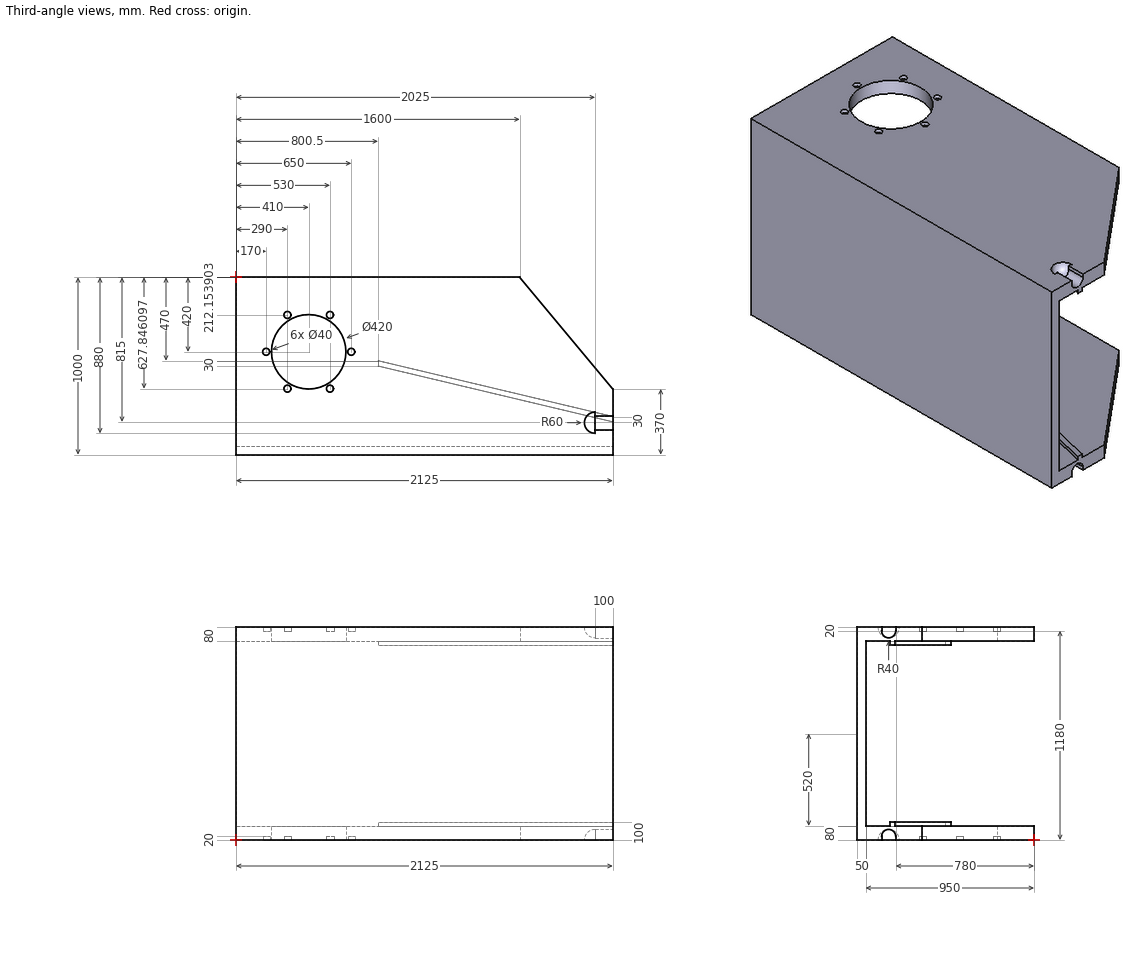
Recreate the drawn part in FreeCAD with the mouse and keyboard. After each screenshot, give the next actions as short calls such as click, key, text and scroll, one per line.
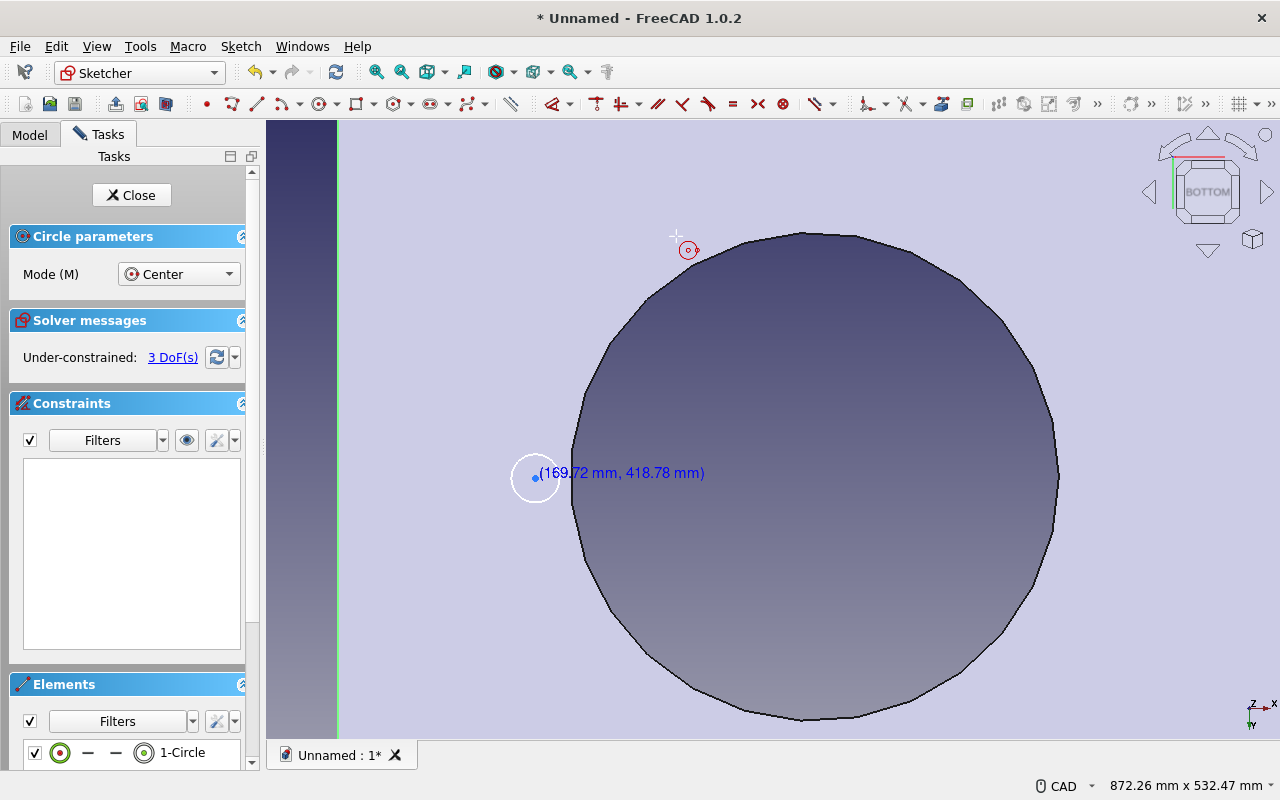
click(675, 235)
click(692, 219)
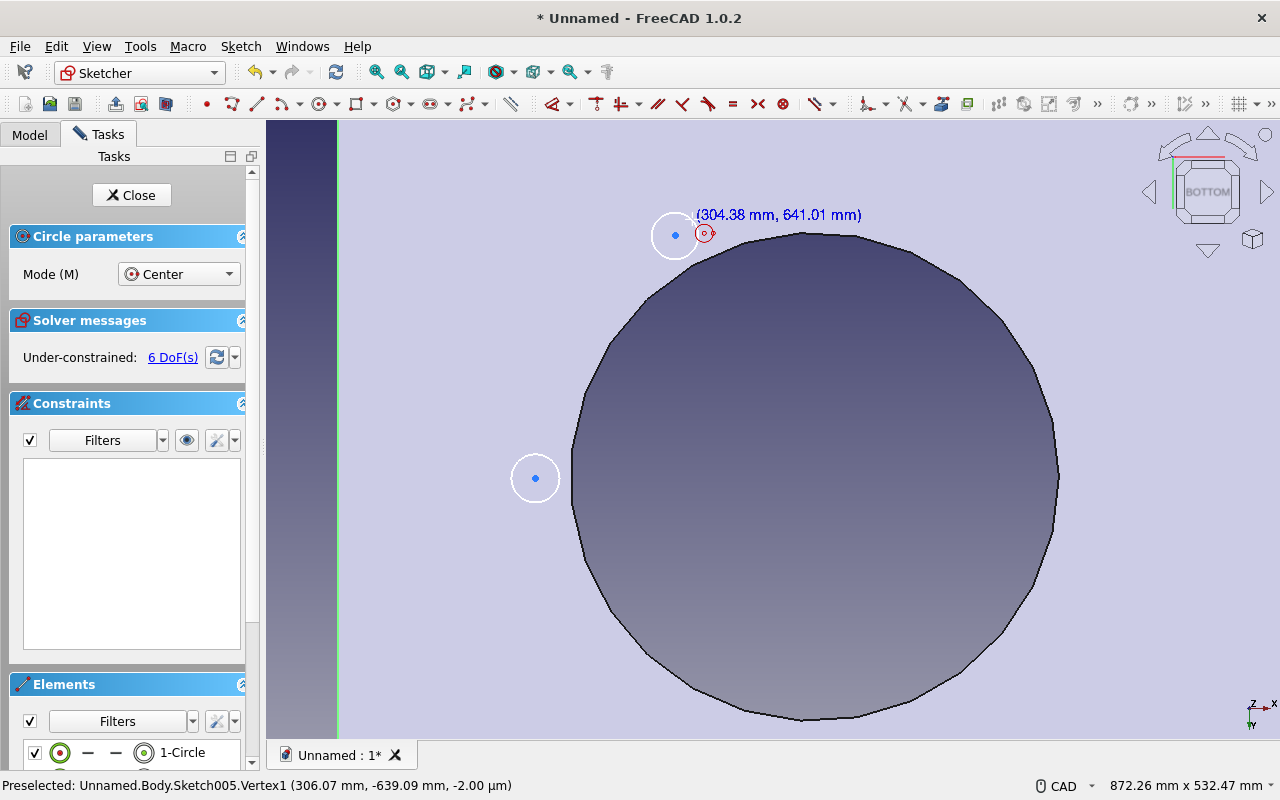
click(954, 235)
click(971, 219)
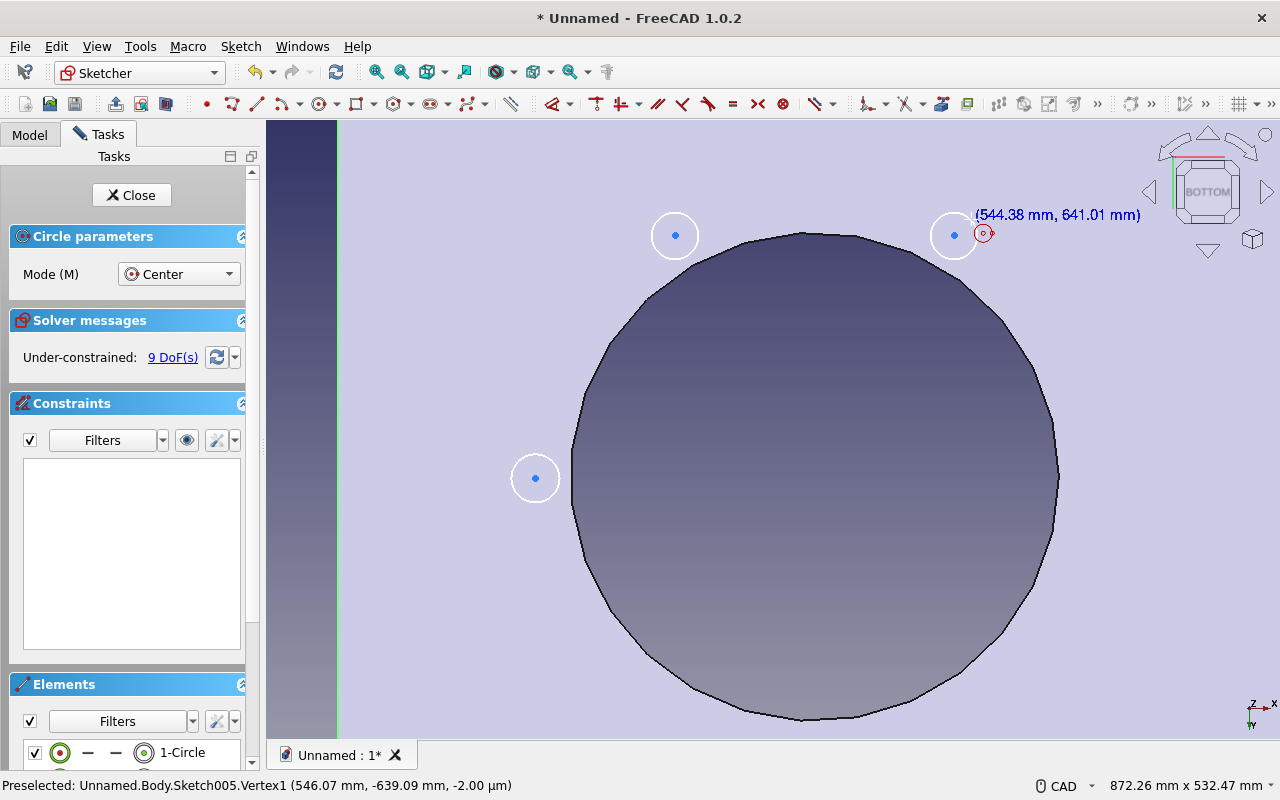
click(1094, 477)
click(1110, 460)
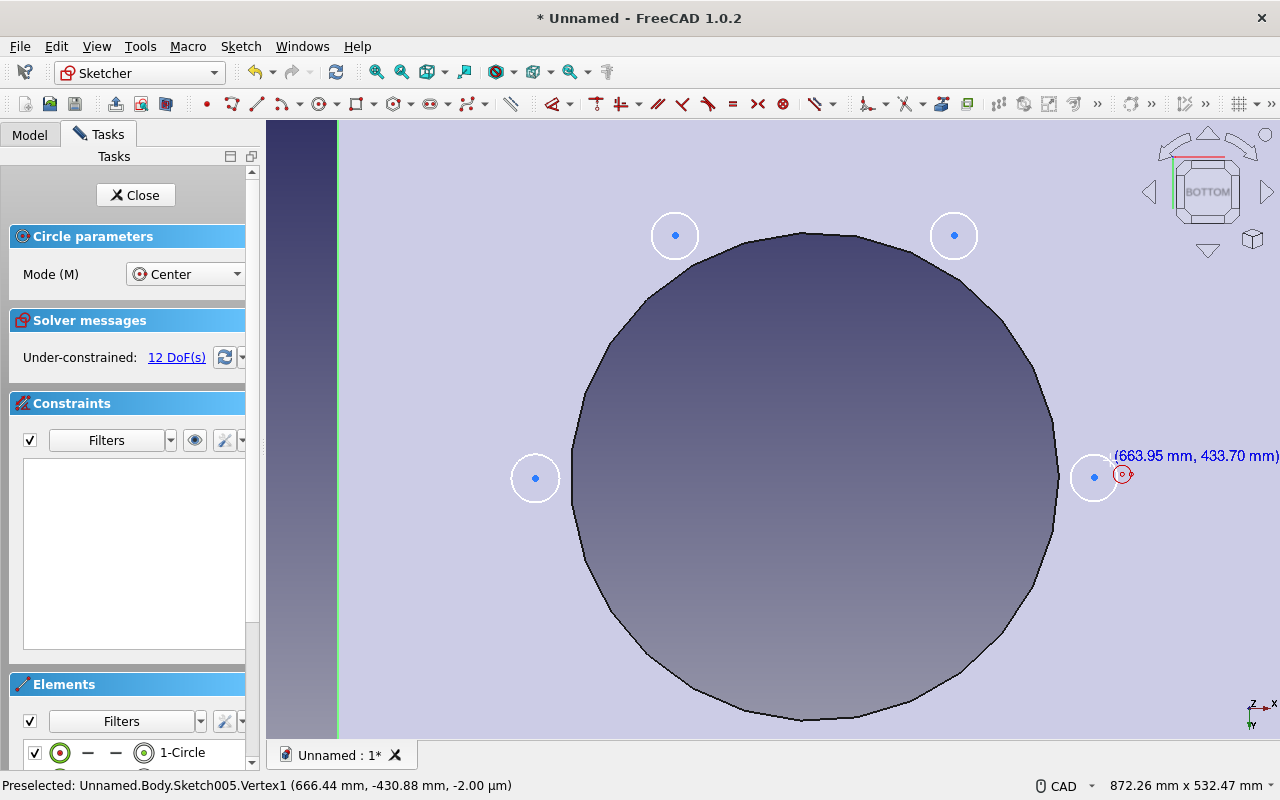
scroll(676, 236, down, 3)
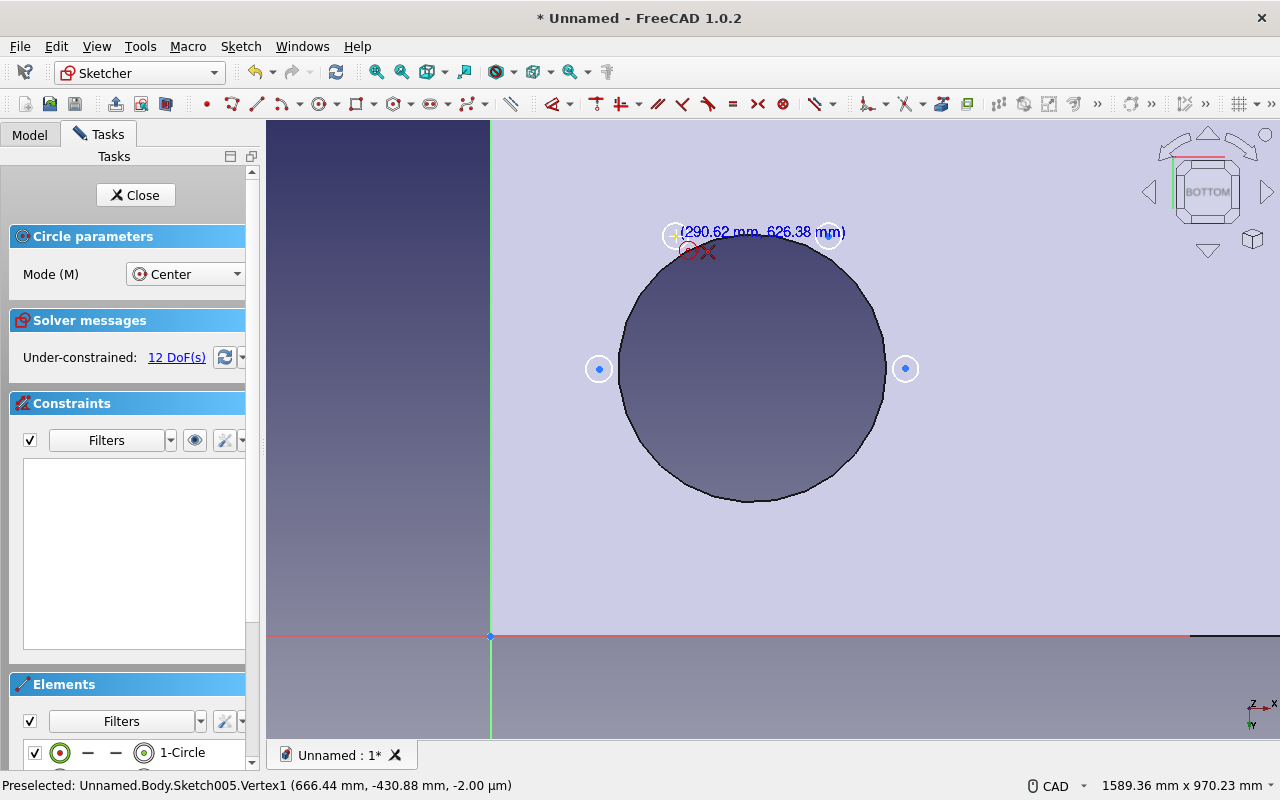
scroll(676, 501, up, 3)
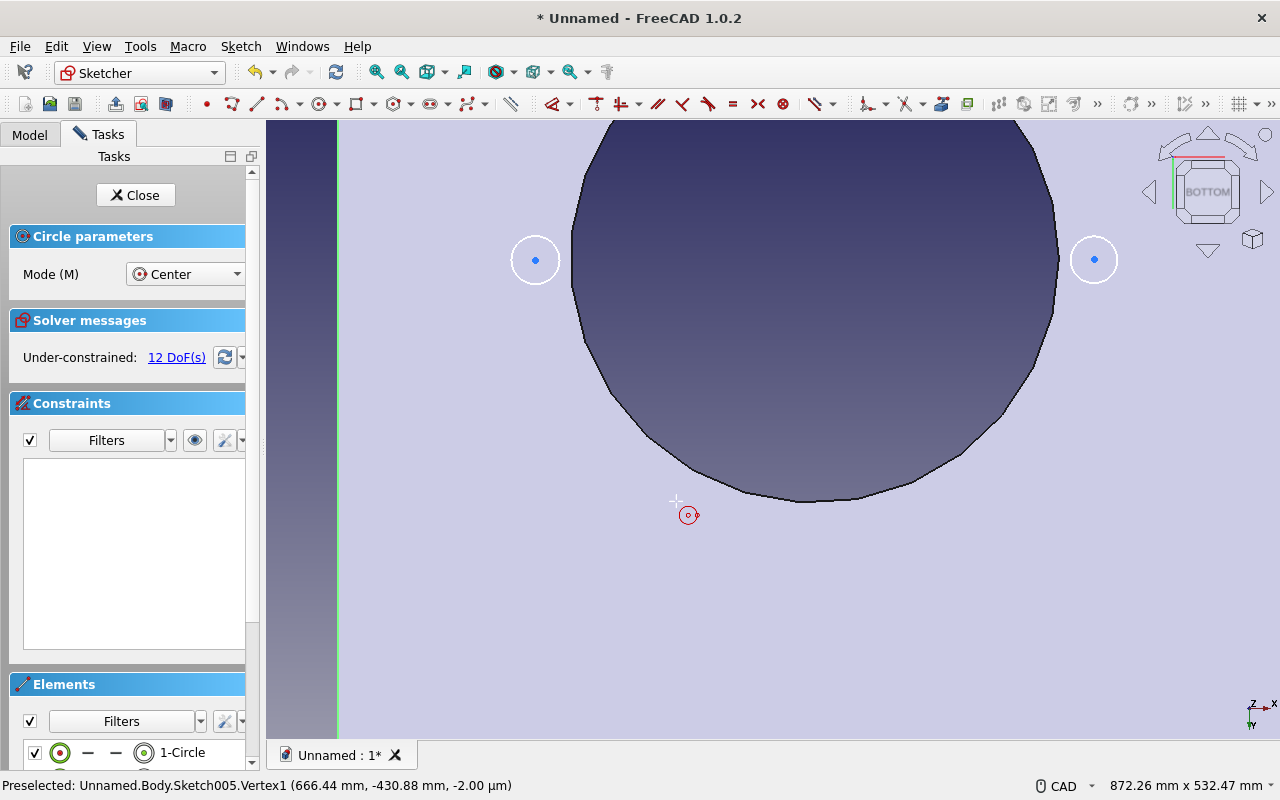
click(675, 500)
click(692, 484)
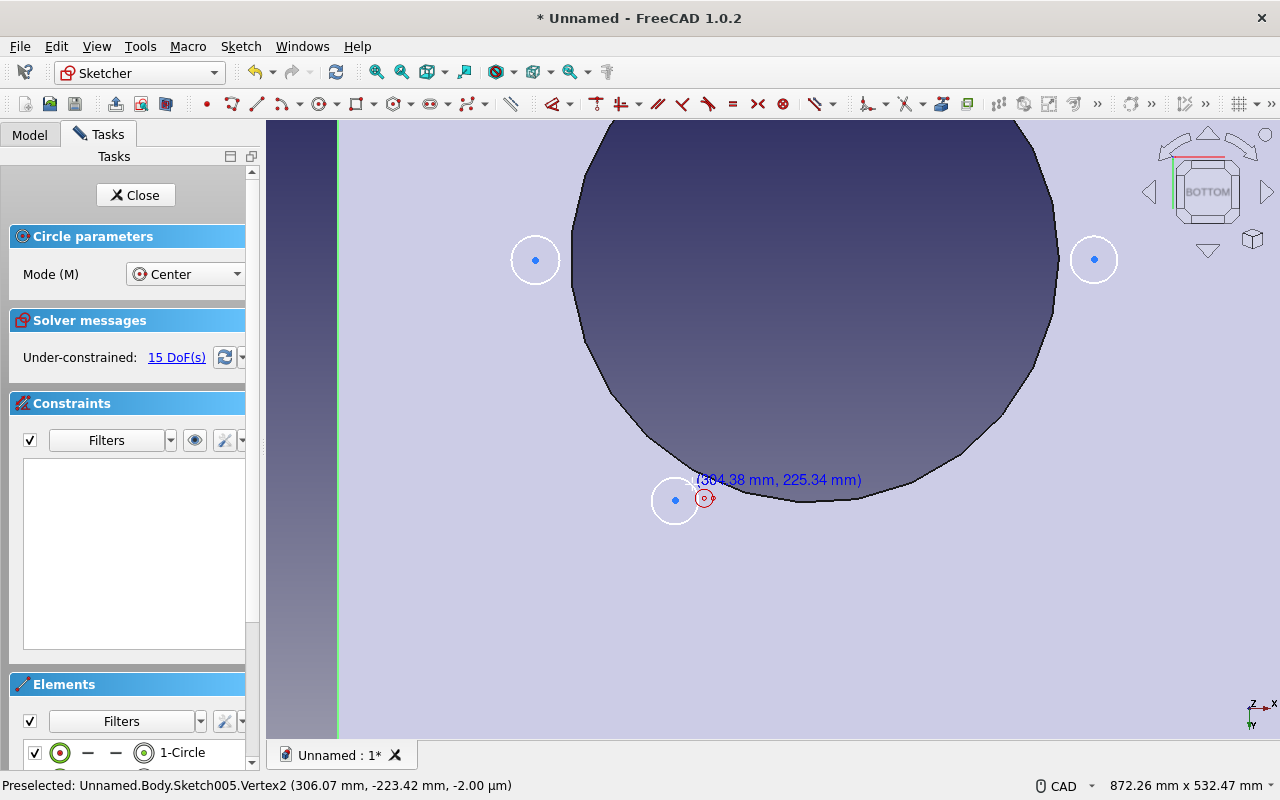
click(954, 500)
click(971, 484)
key(Escape)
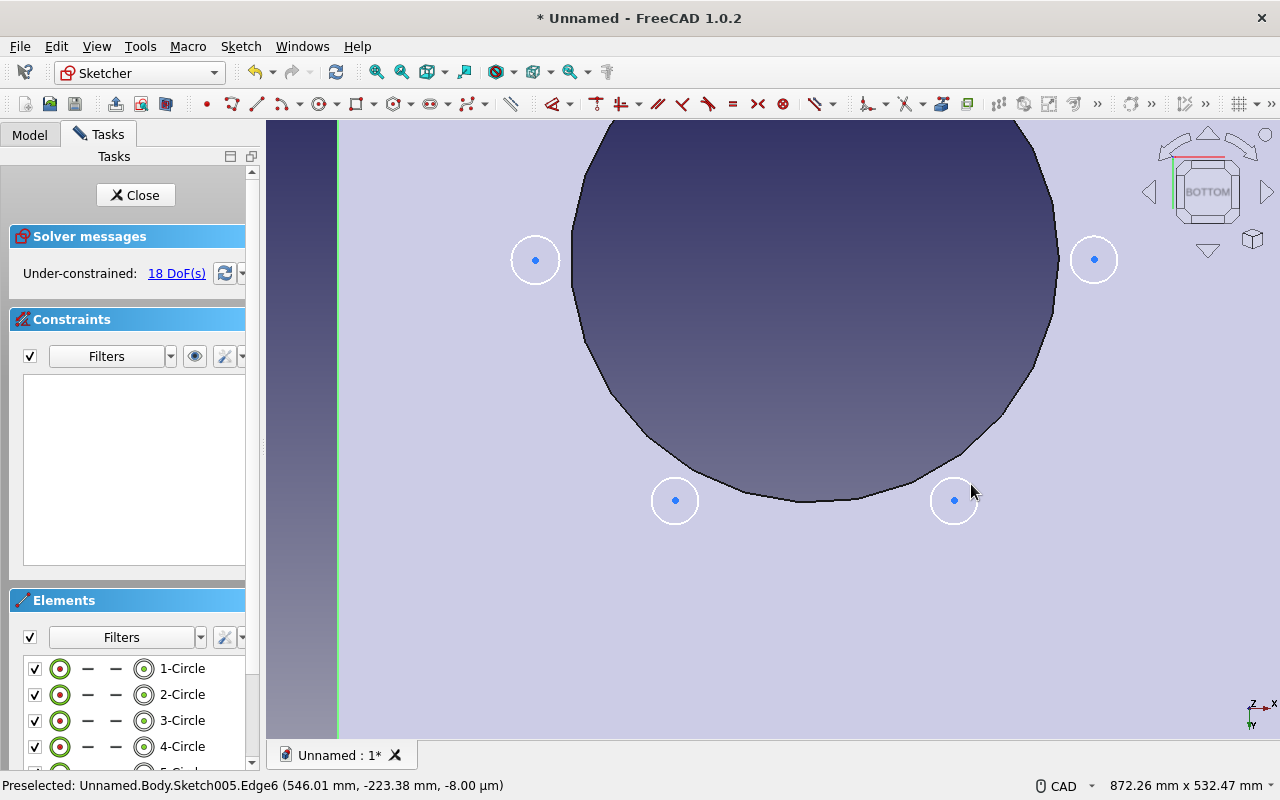
click(552, 243)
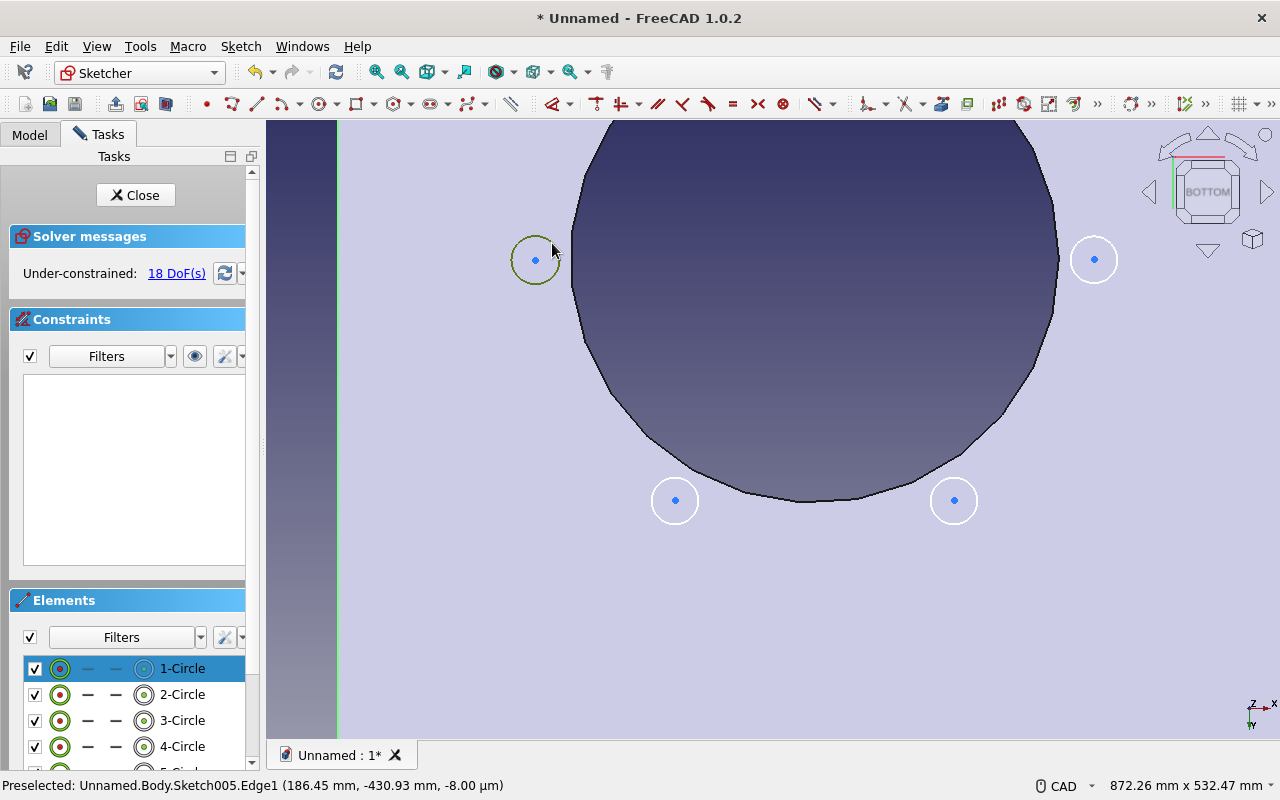
scroll(676, 501, down, 3)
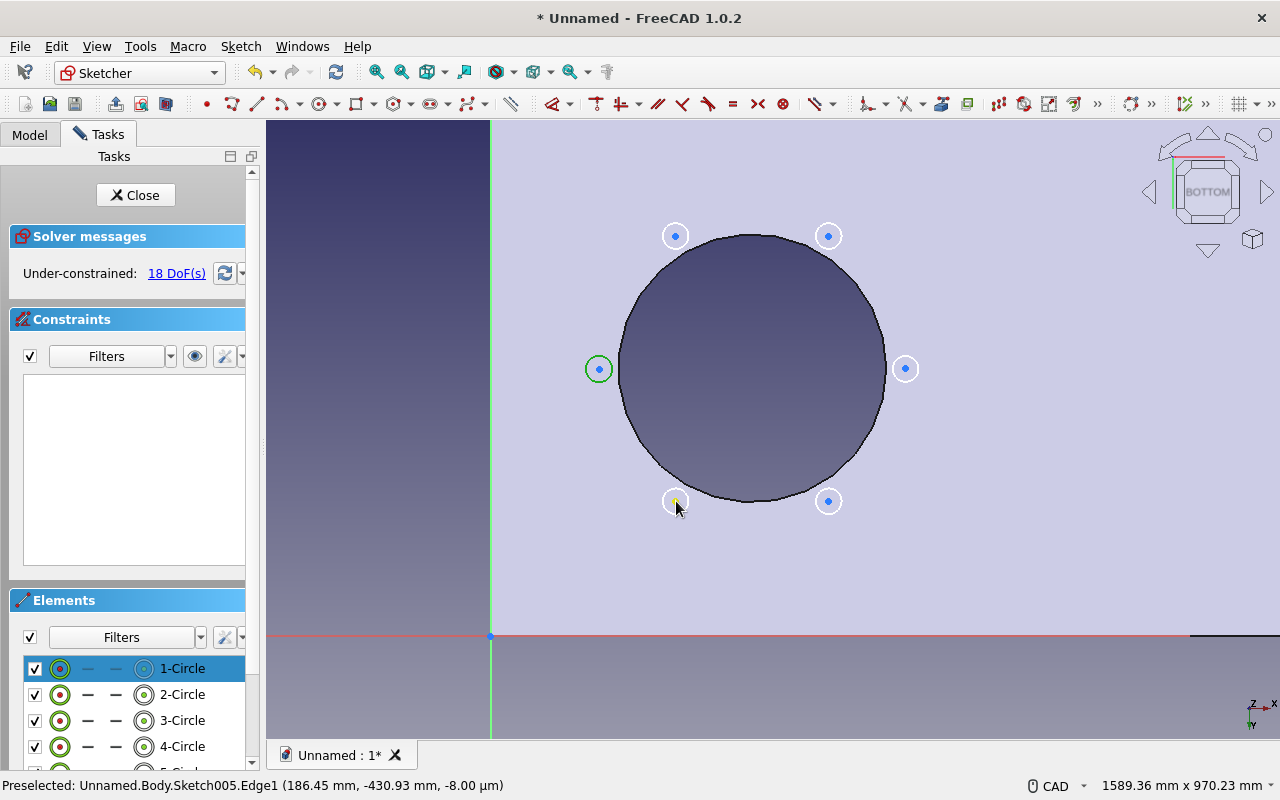
click(685, 227)